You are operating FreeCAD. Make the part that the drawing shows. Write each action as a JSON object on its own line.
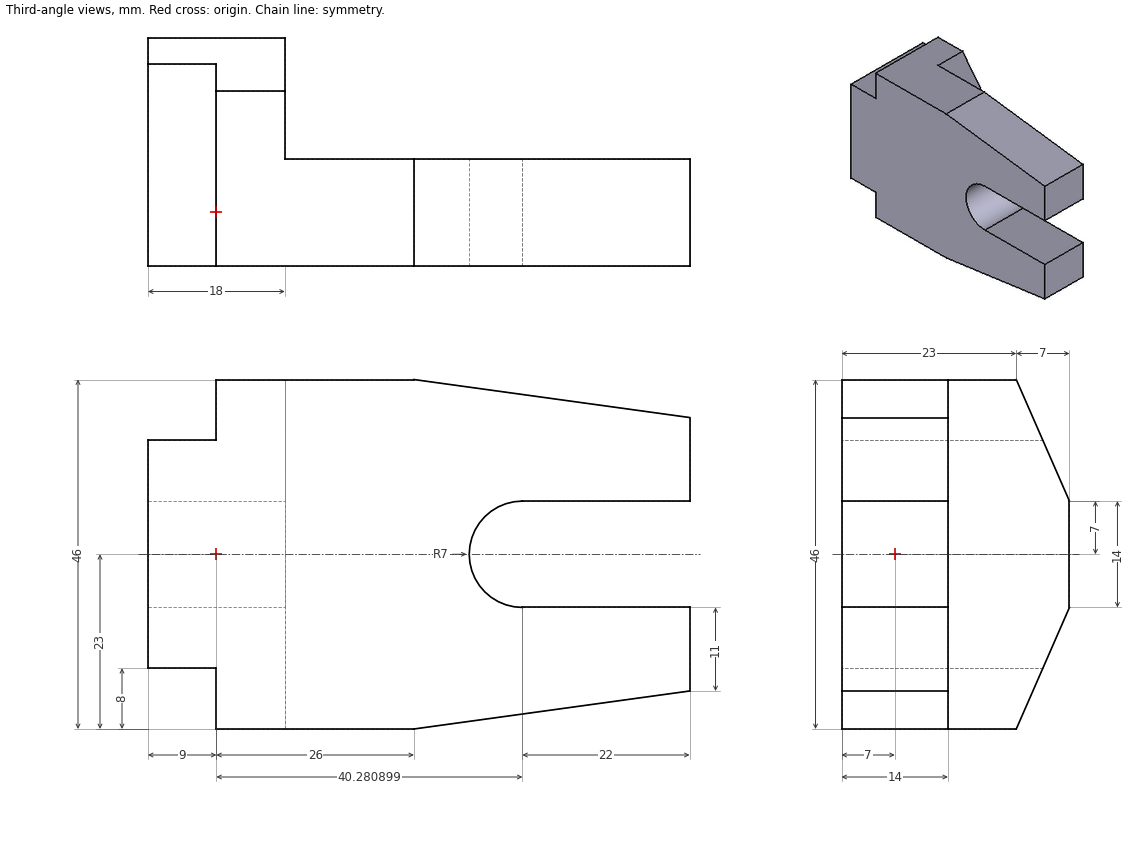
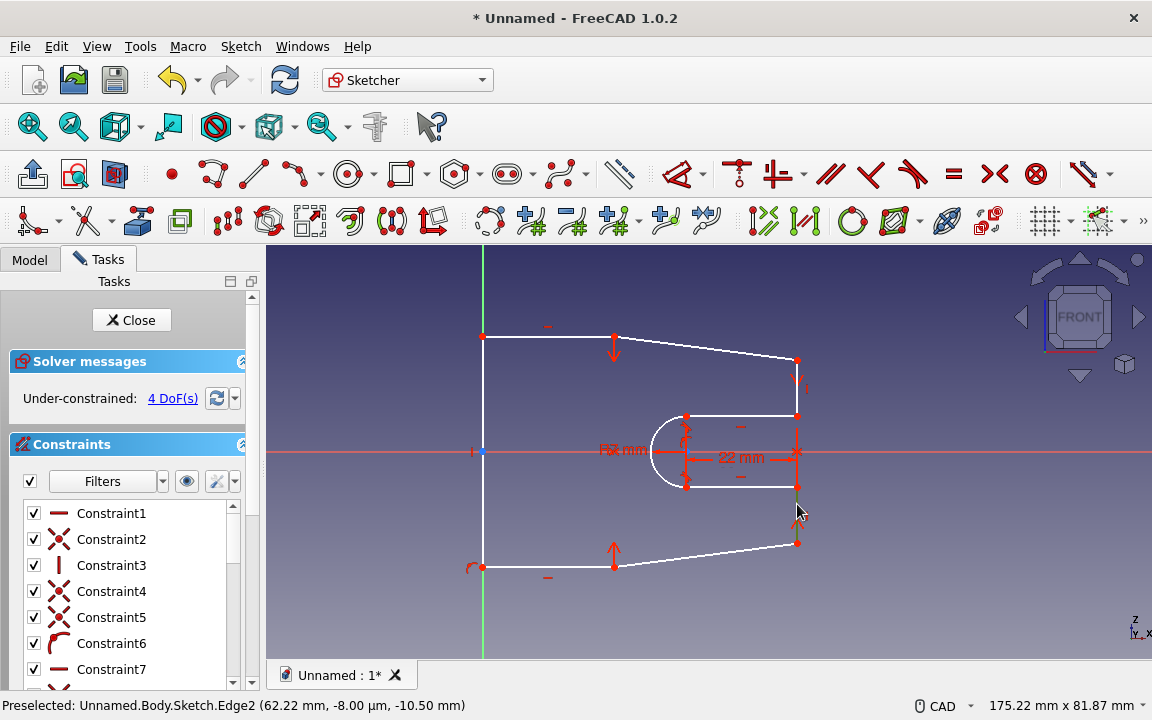
{"action": "key", "text": "i"}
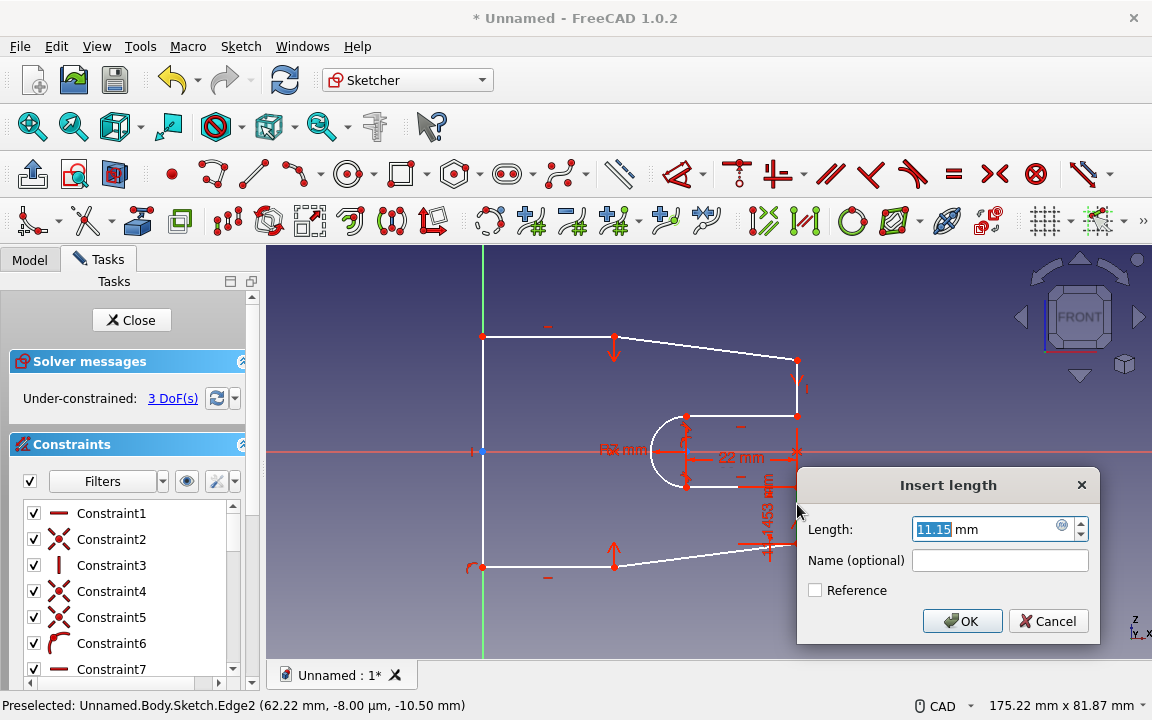
{"action": "type", "text": "11"}
{"action": "key", "text": "Return"}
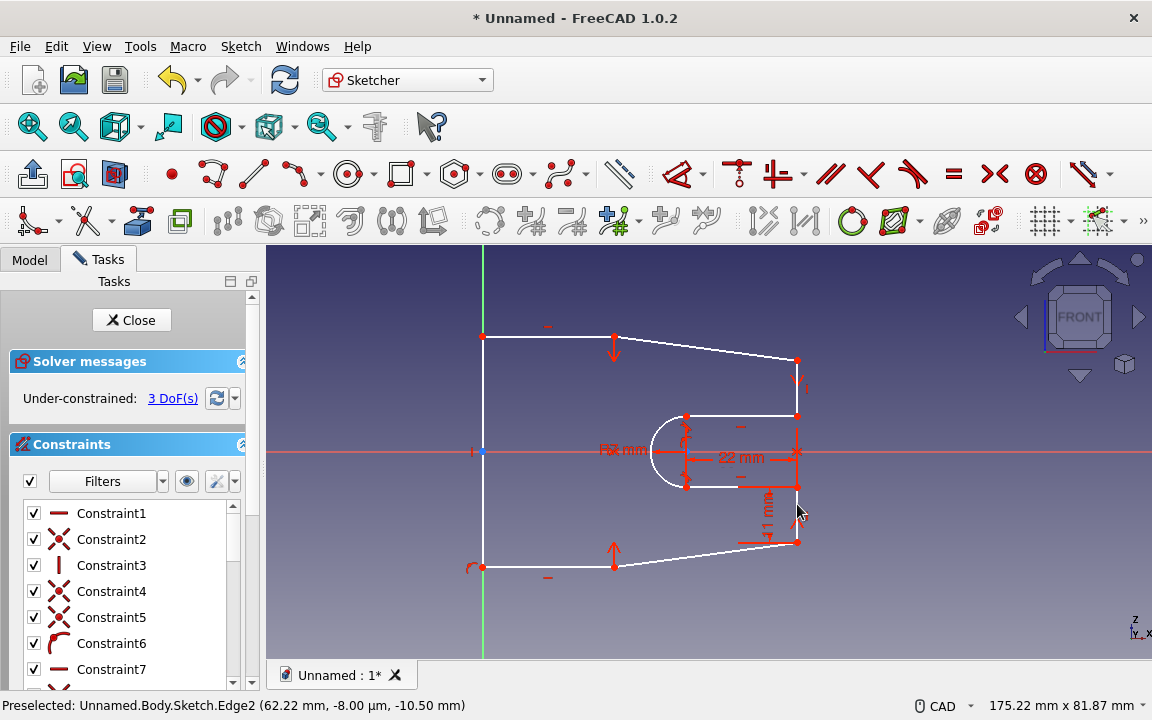
{"action": "left_click", "coordinate": [575, 567]}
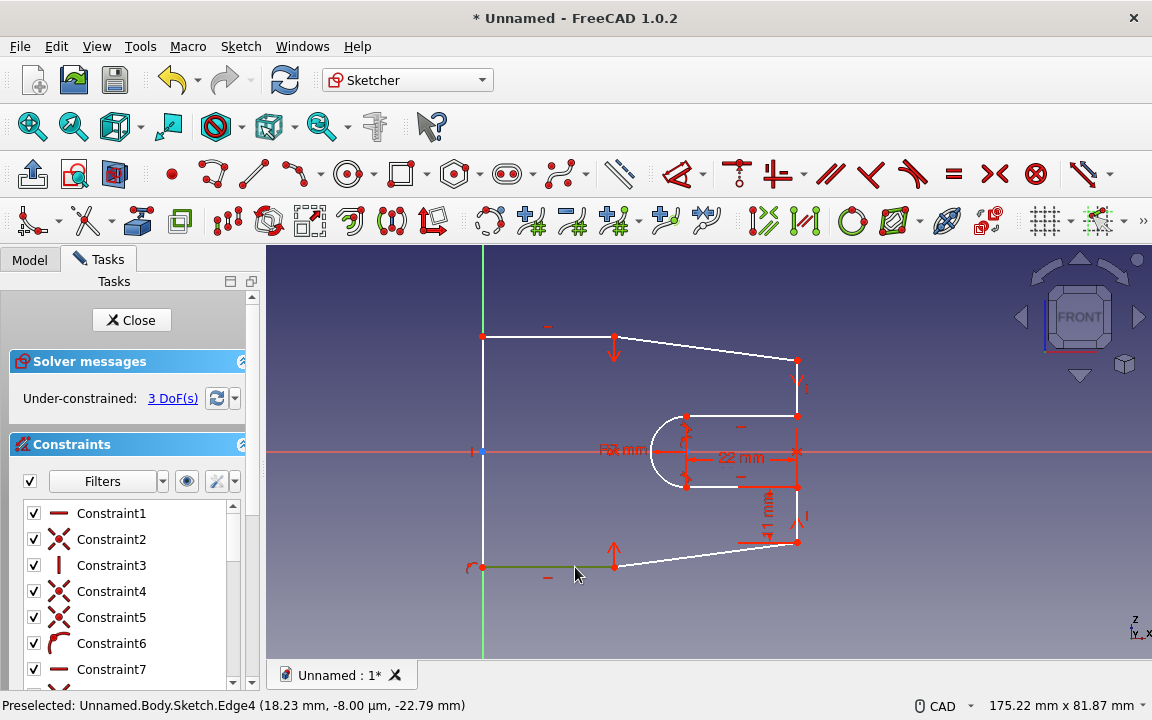
{"action": "key", "text": "l"}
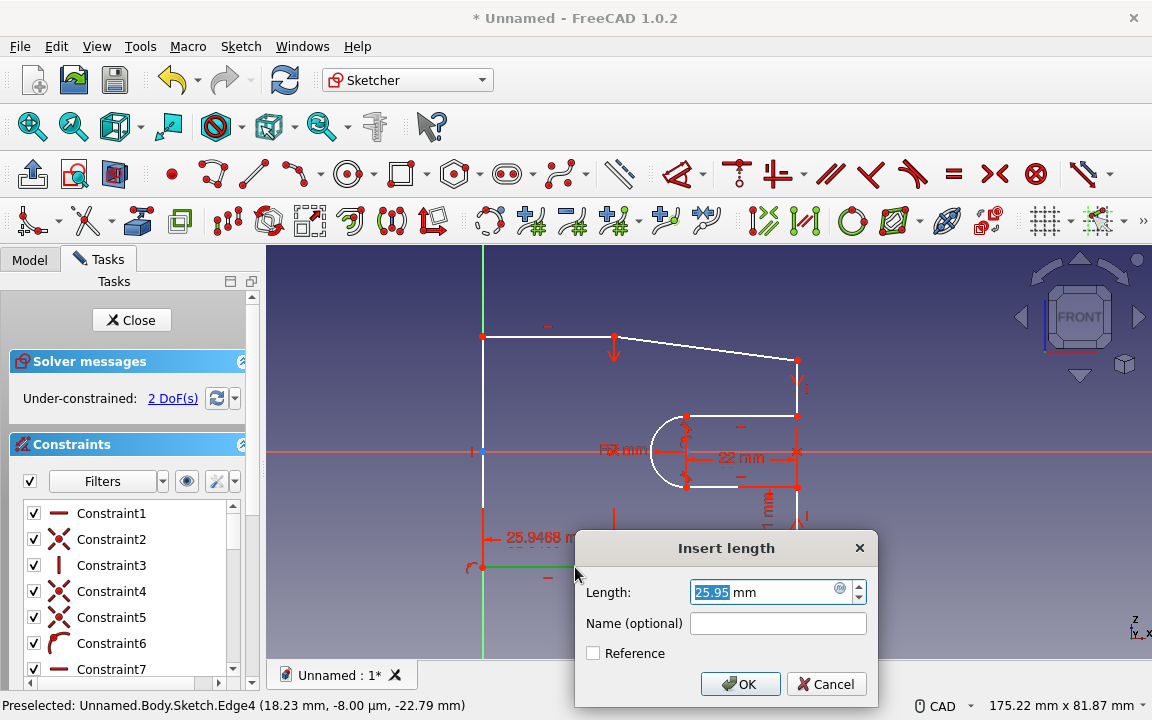
{"action": "type", "text": "26"}
{"action": "key", "text": "Return"}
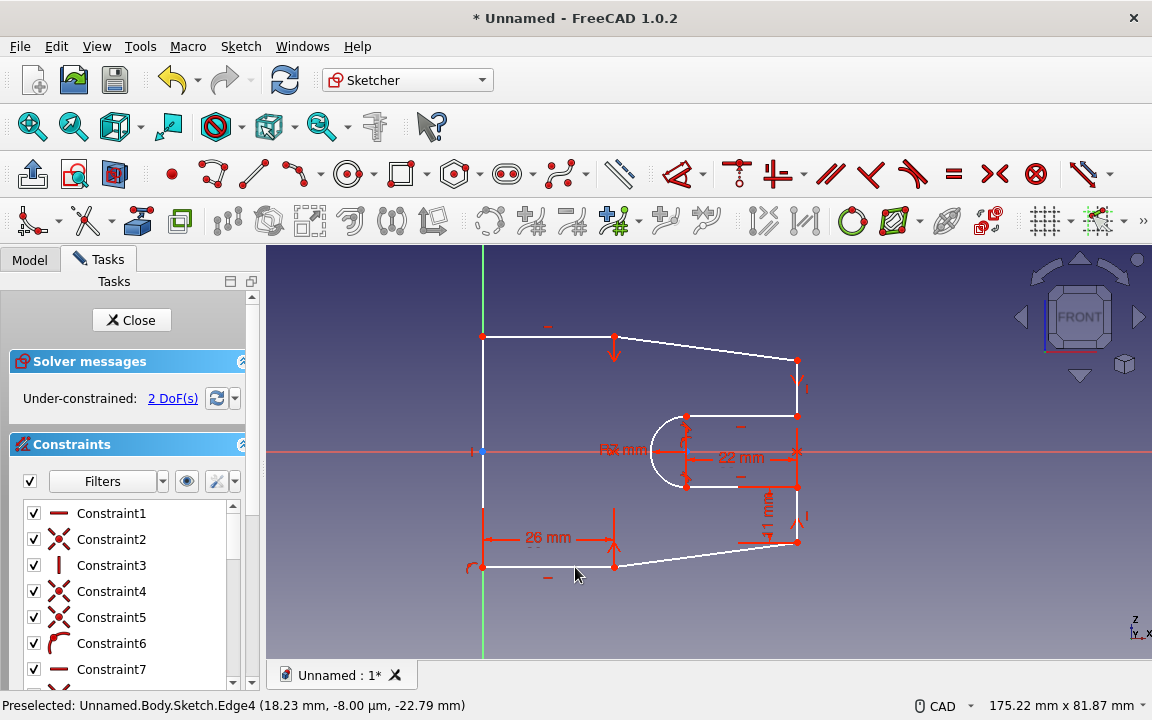
{"action": "left_click", "coordinate": [483, 498]}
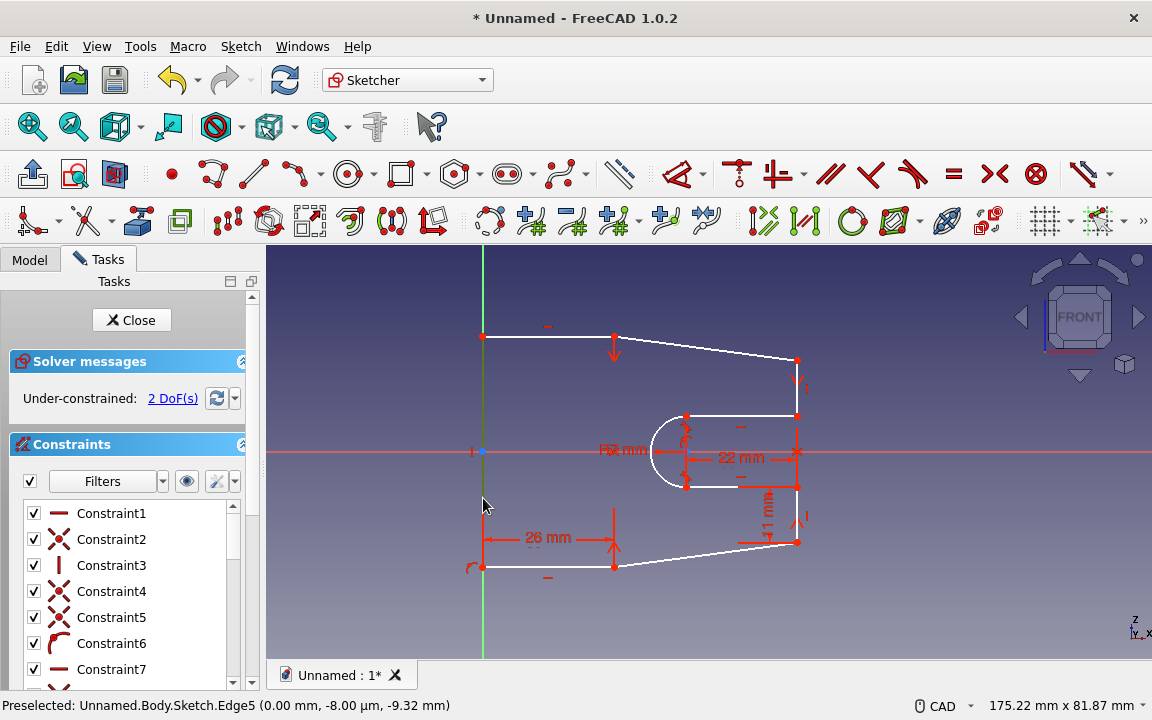
{"action": "key", "text": "i"}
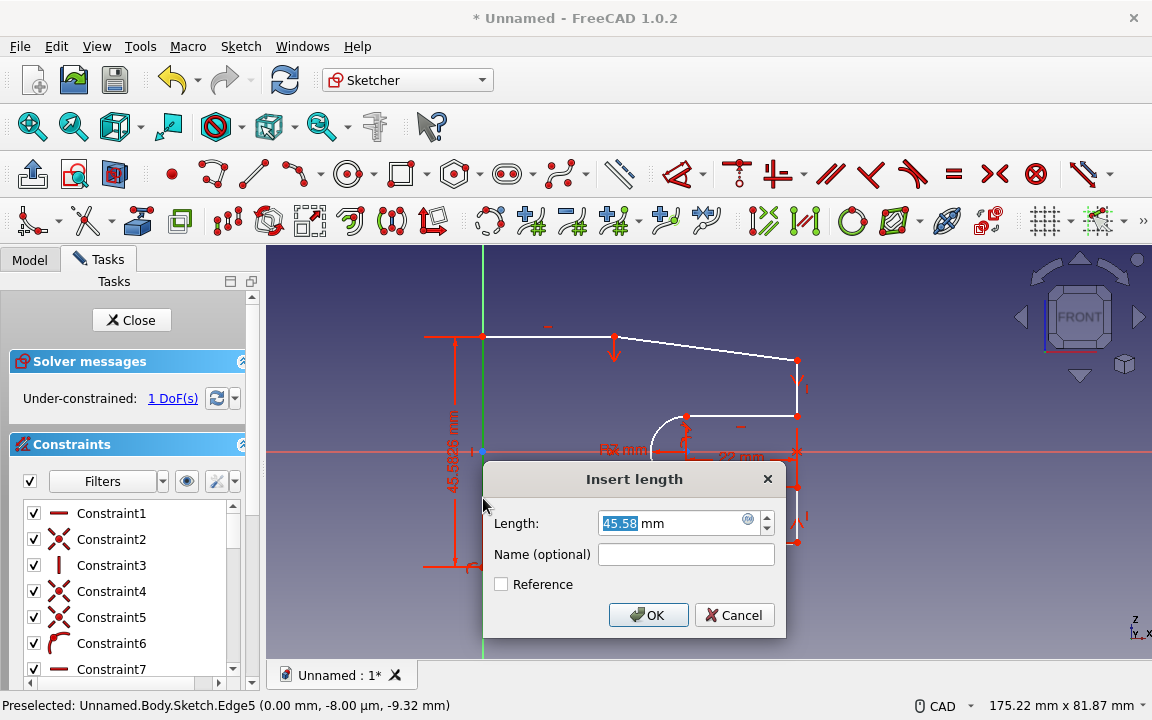
{"action": "type", "text": "46"}
{"action": "key", "text": "Return"}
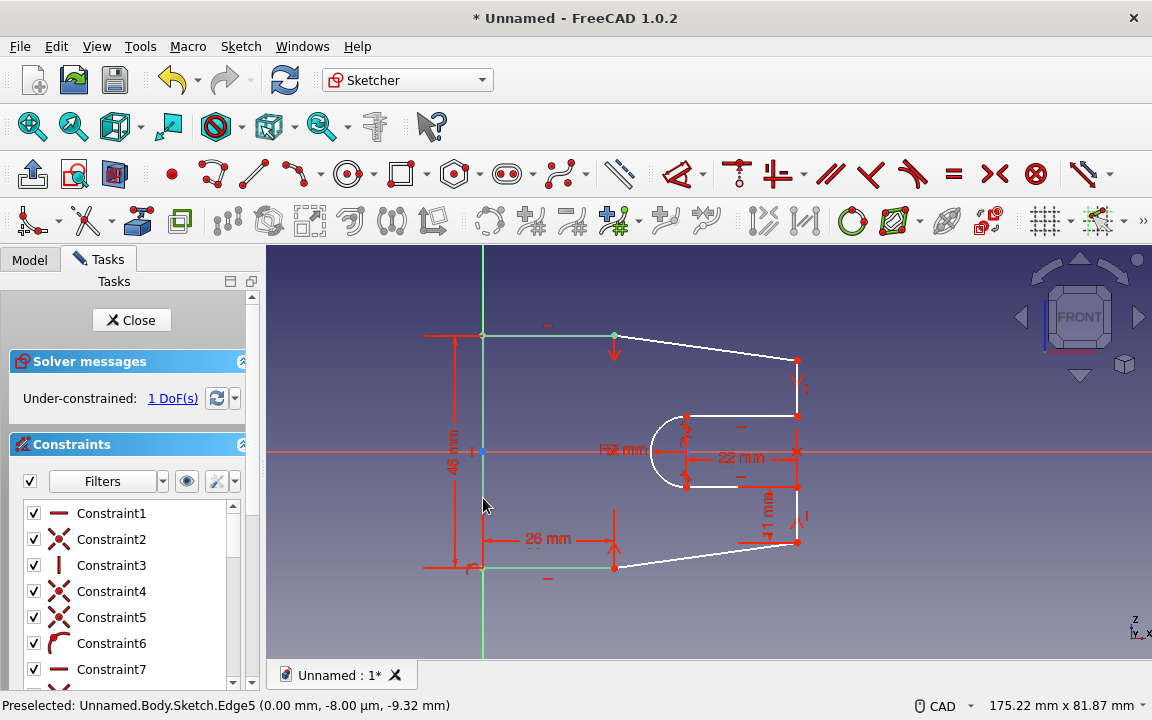
{"action": "left_click", "coordinate": [686, 487]}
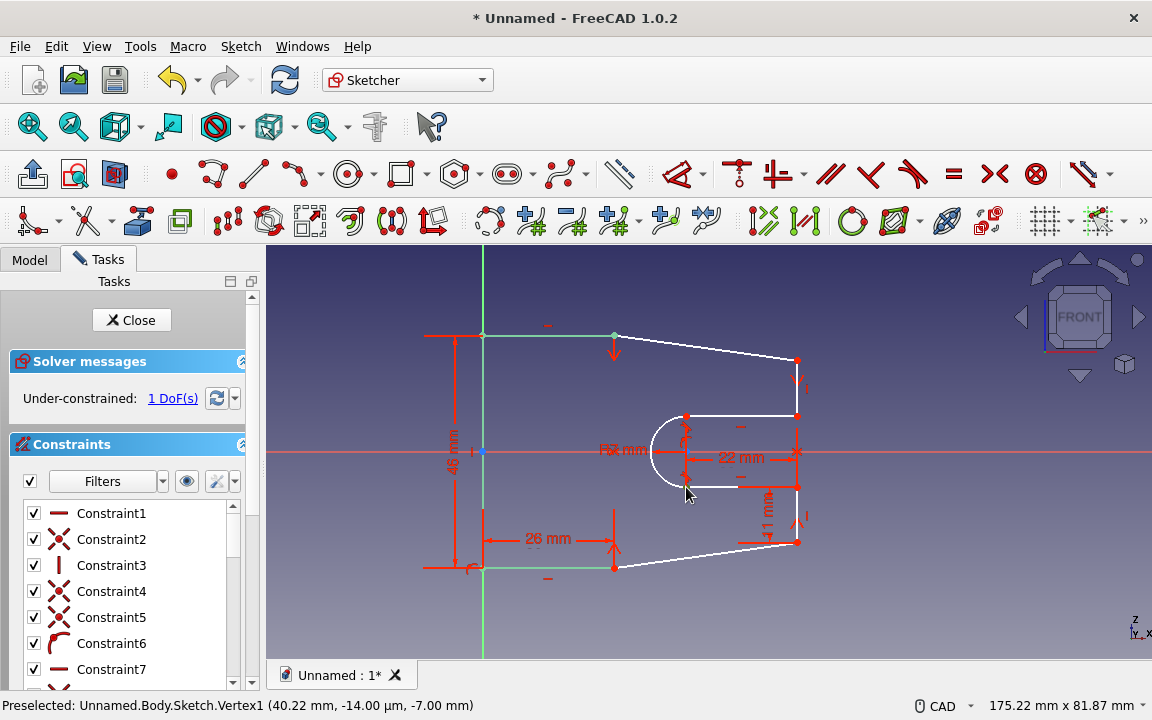
{"action": "key", "text": "l"}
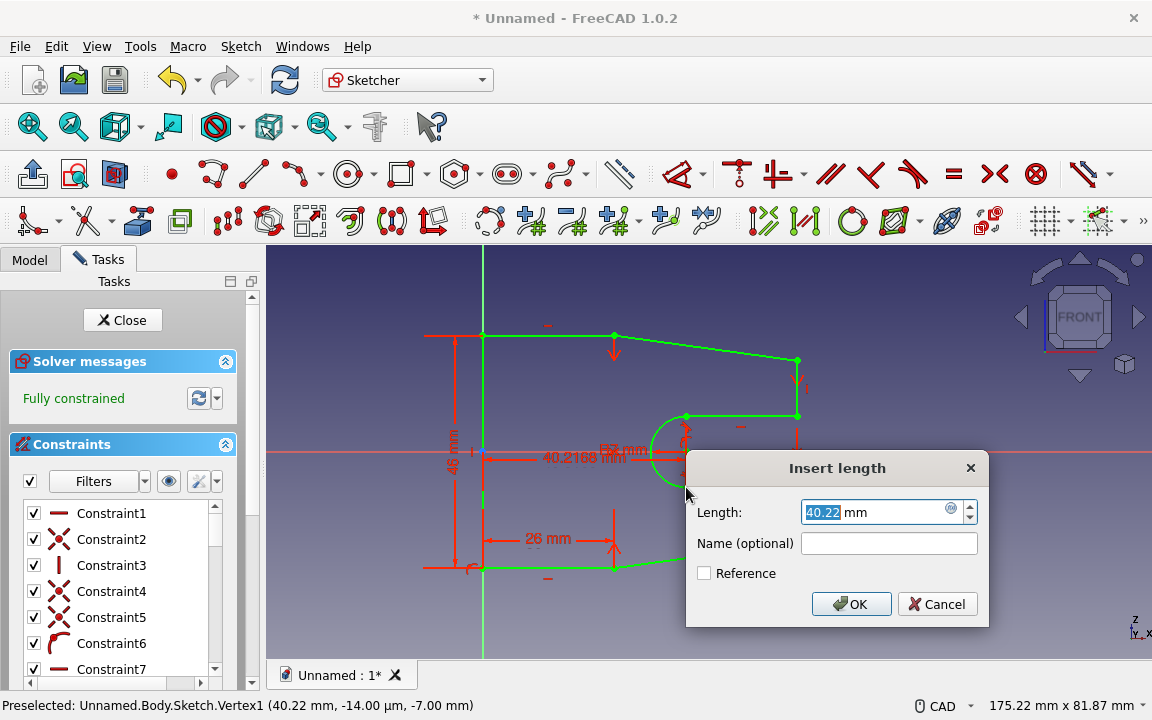
{"action": "type", "text": "40.280899"}
{"action": "key", "text": "Return"}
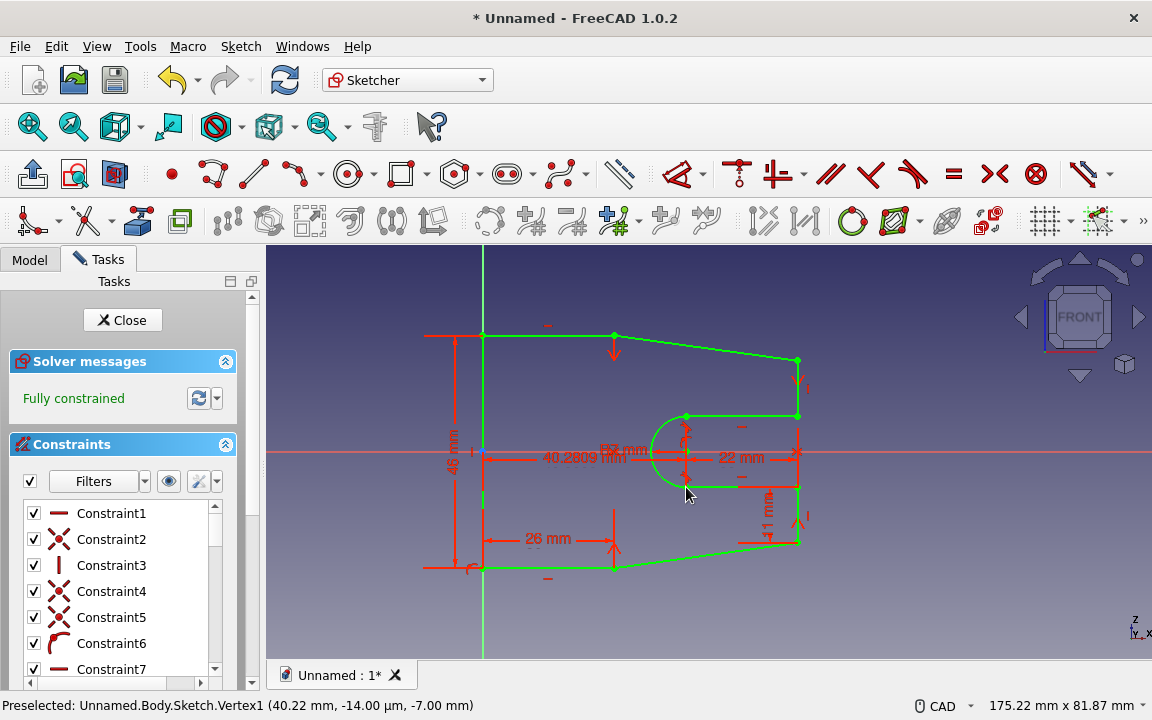
{"action": "left_click", "coordinate": [123, 320]}